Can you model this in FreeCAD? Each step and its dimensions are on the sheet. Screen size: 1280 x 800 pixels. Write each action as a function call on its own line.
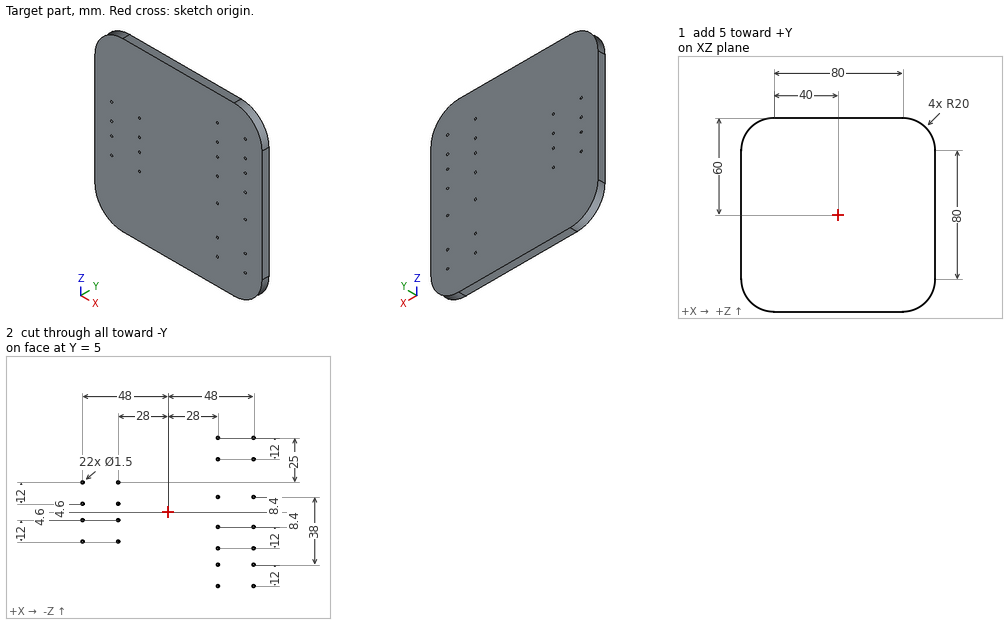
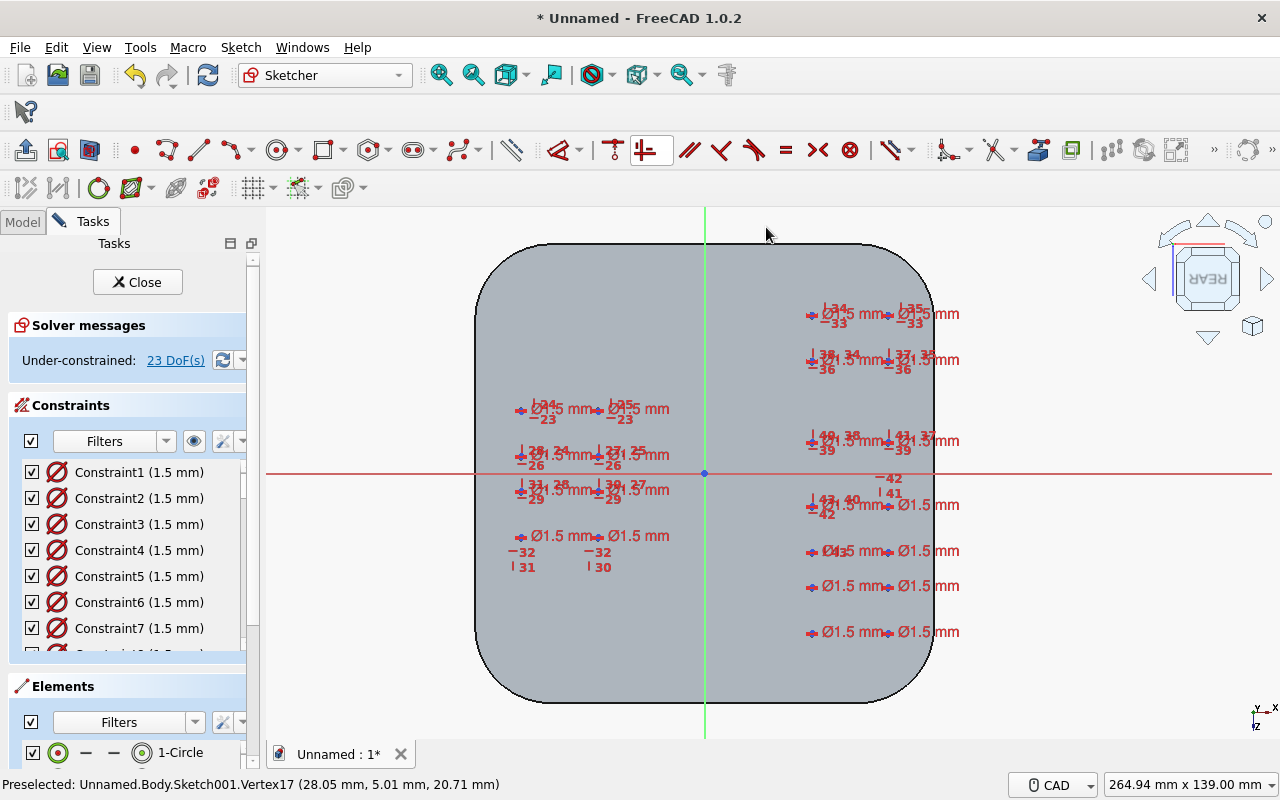
click(888, 507)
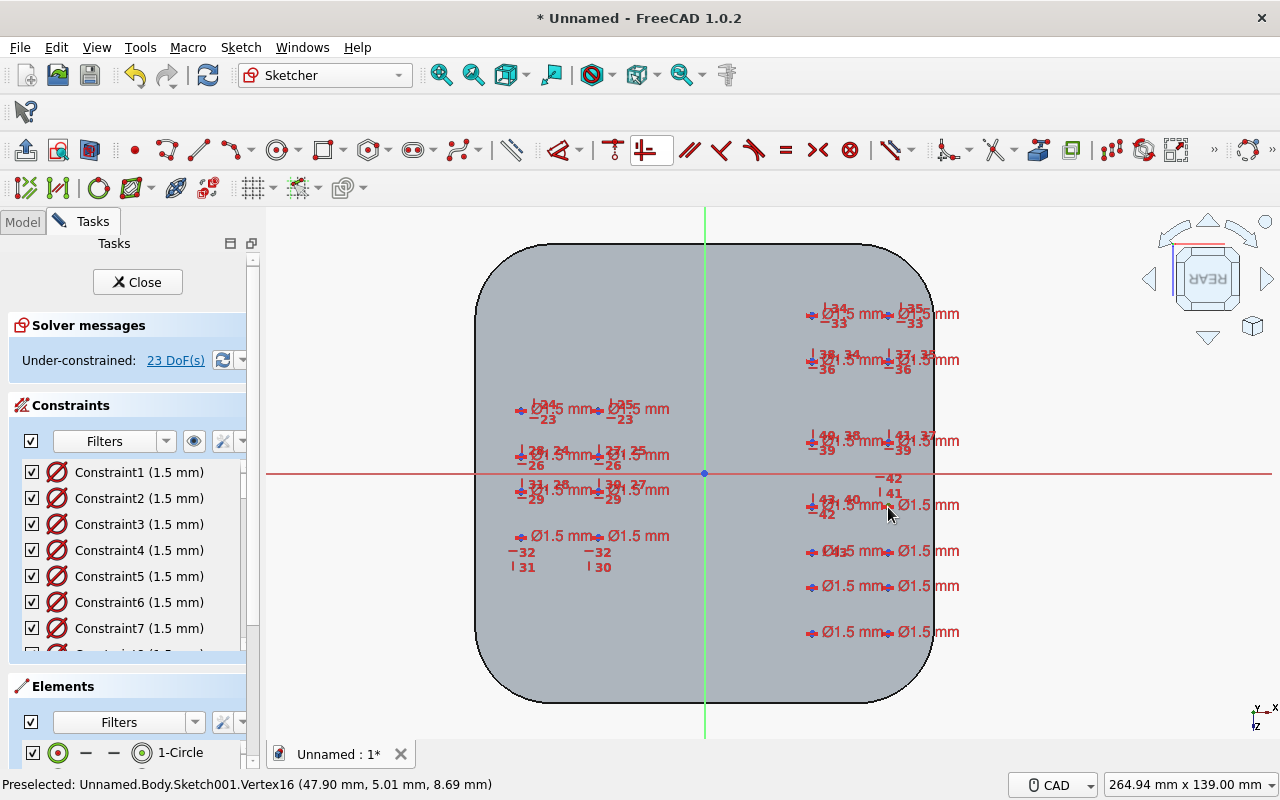
click(888, 553)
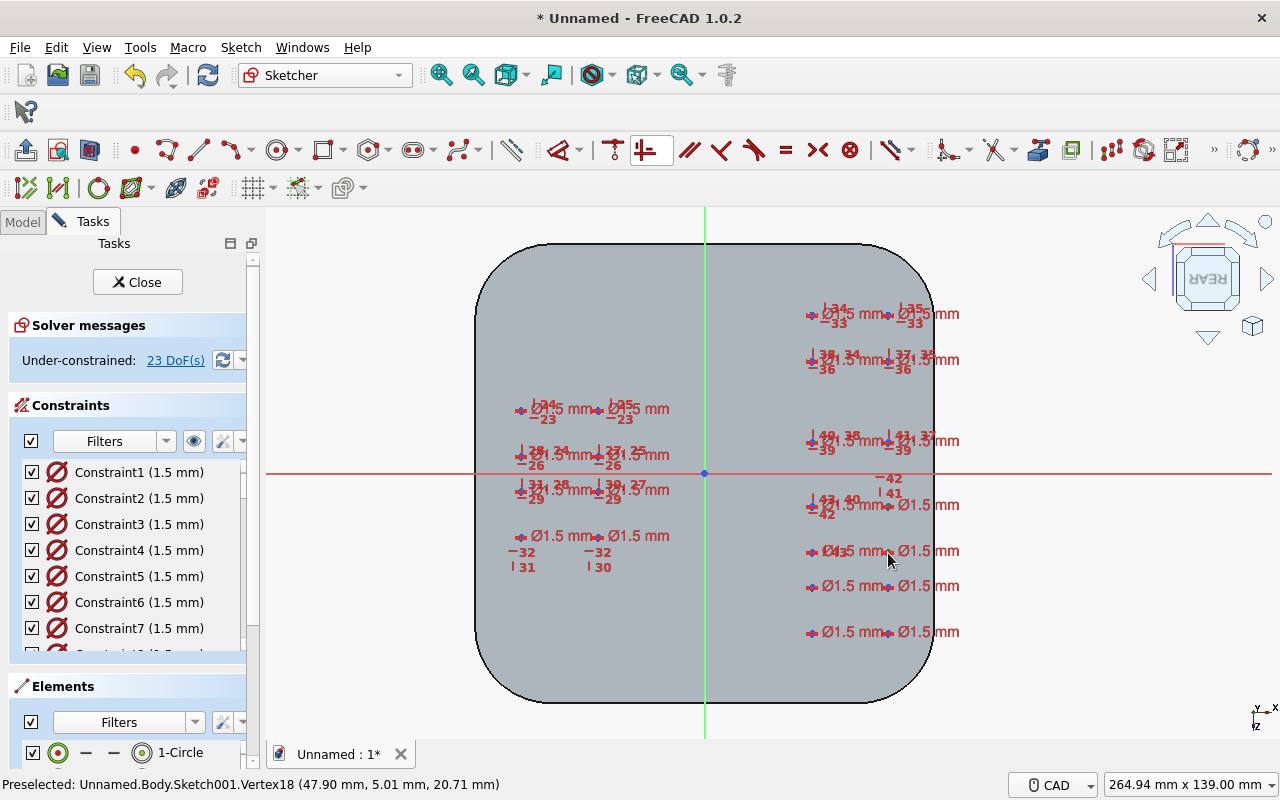
key(v)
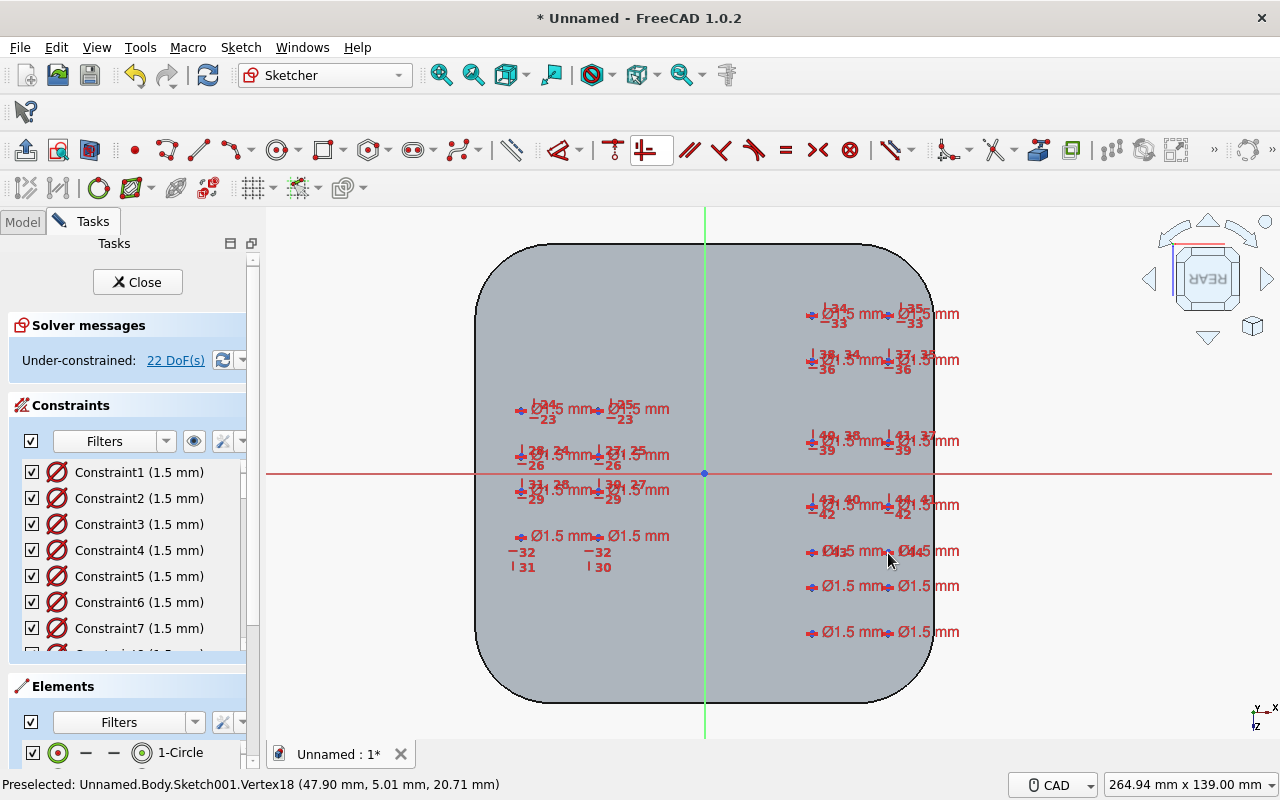
click(812, 553)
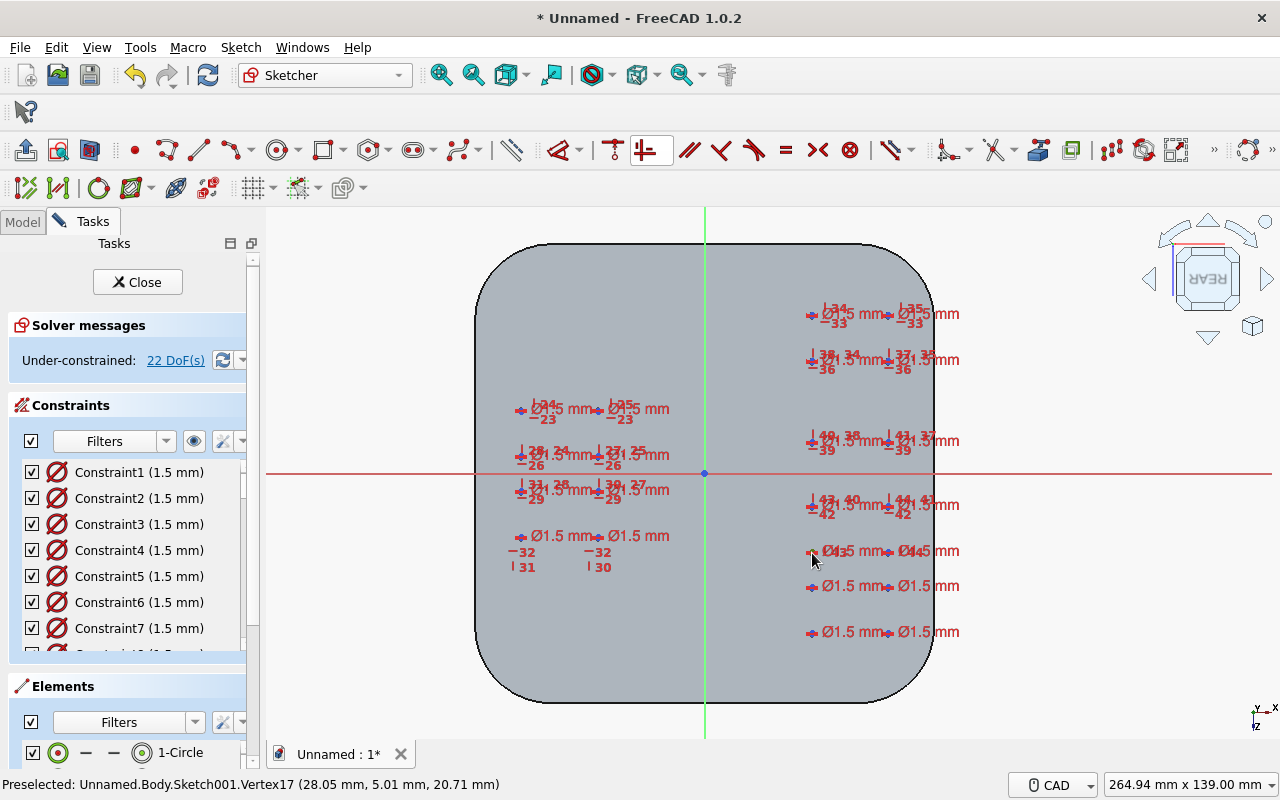
click(888, 553)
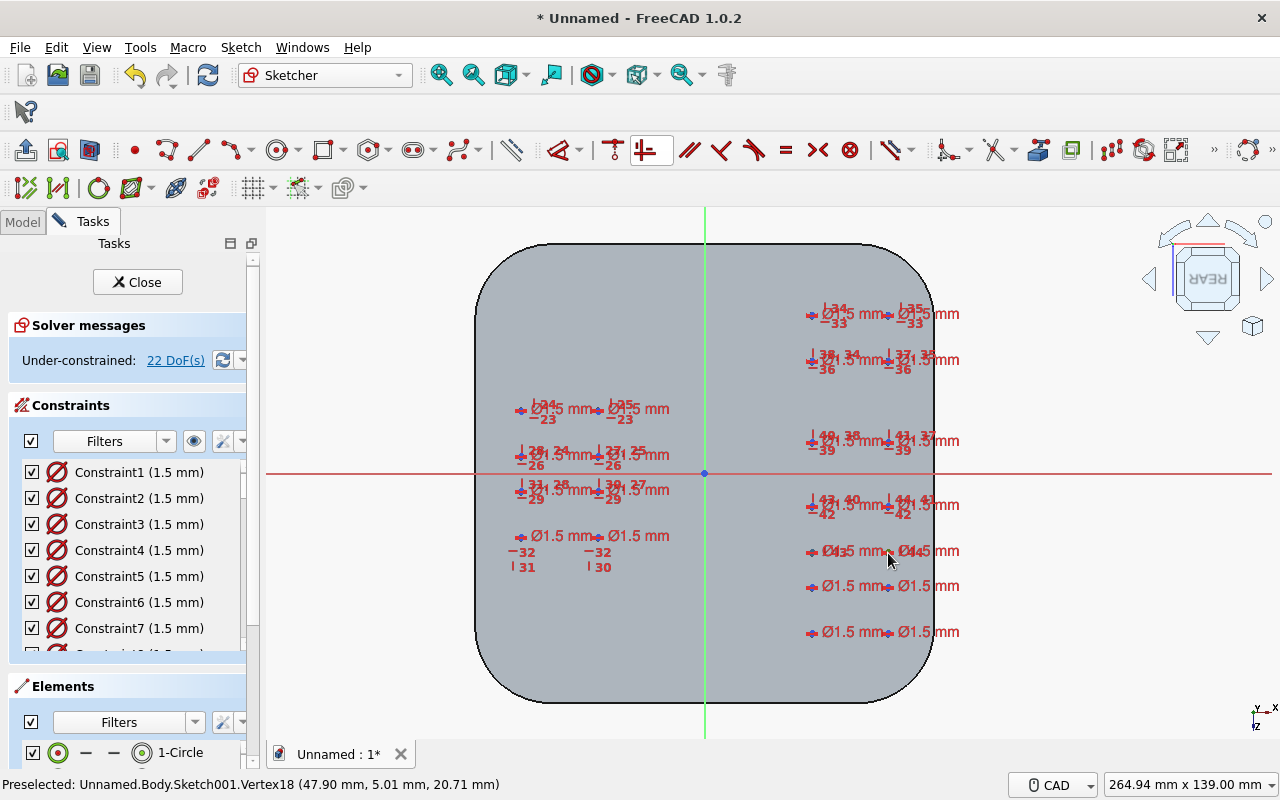
key(h)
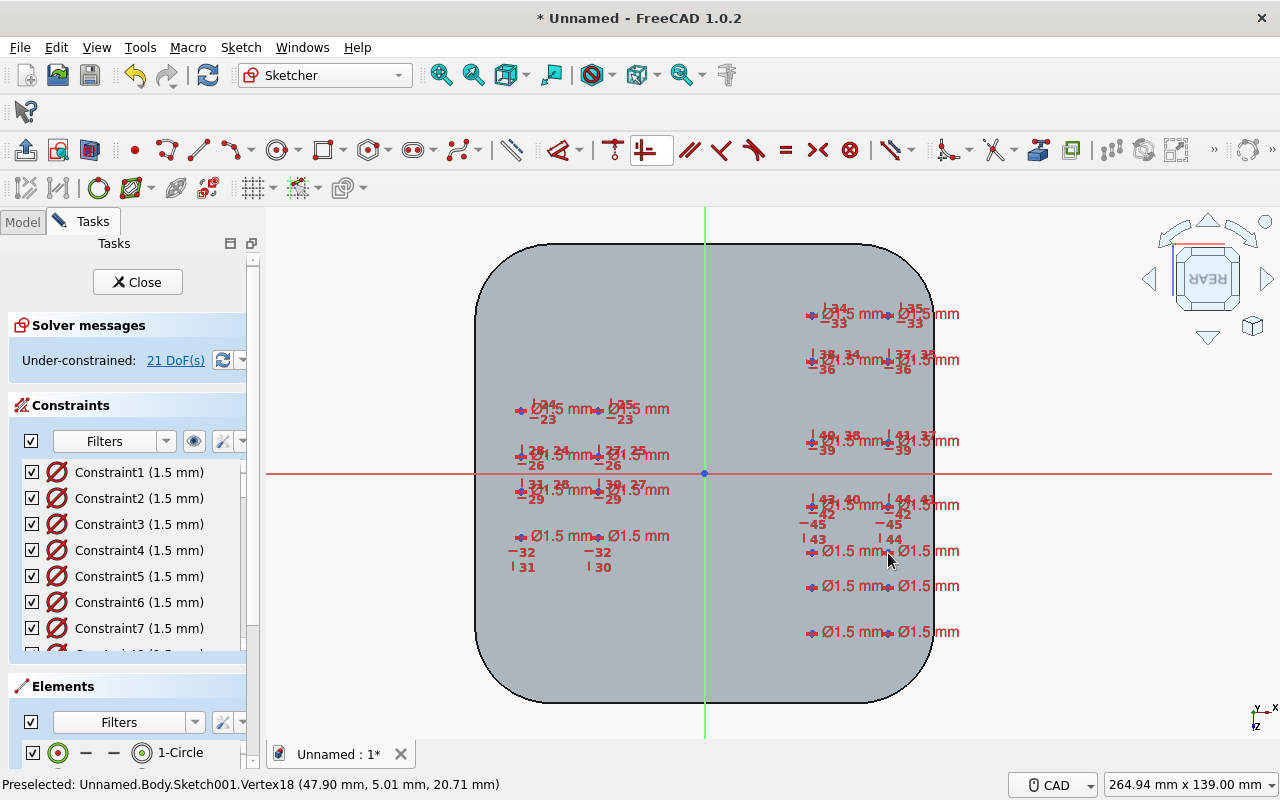
click(888, 553)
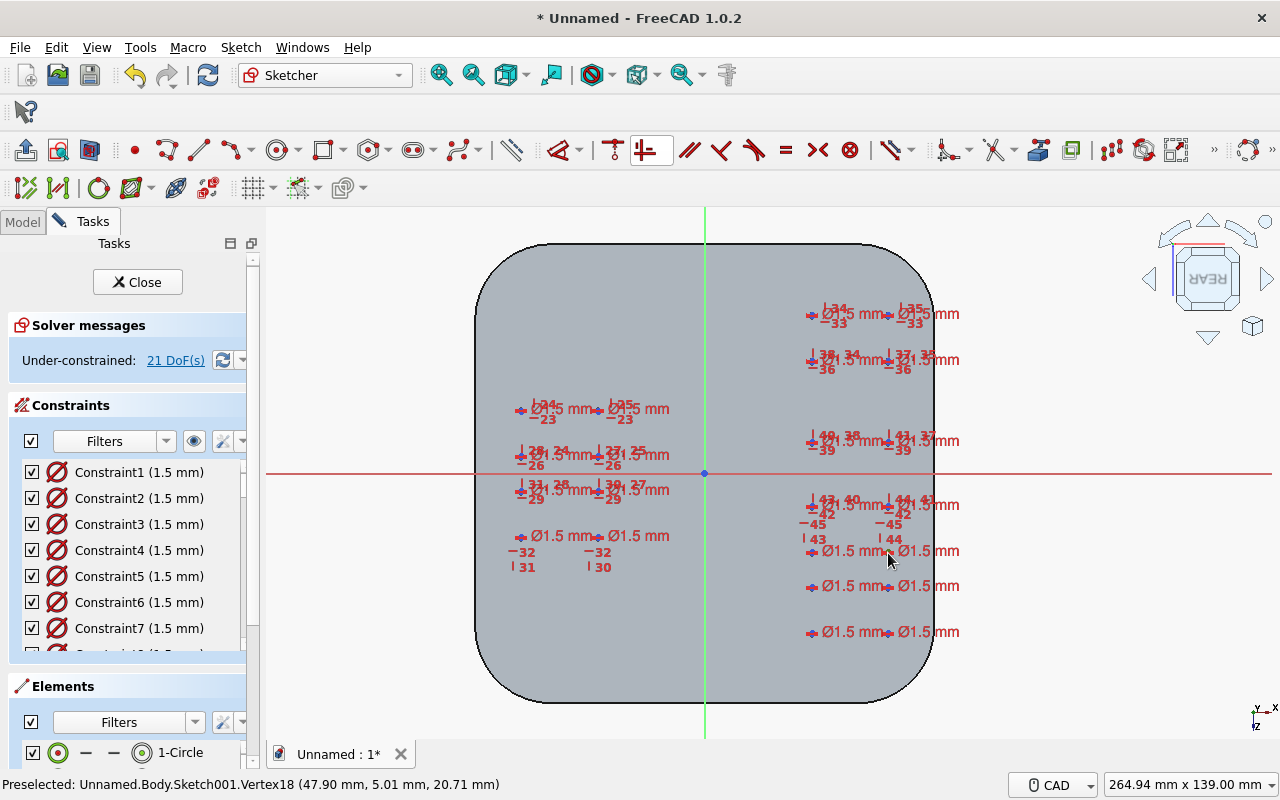
click(888, 588)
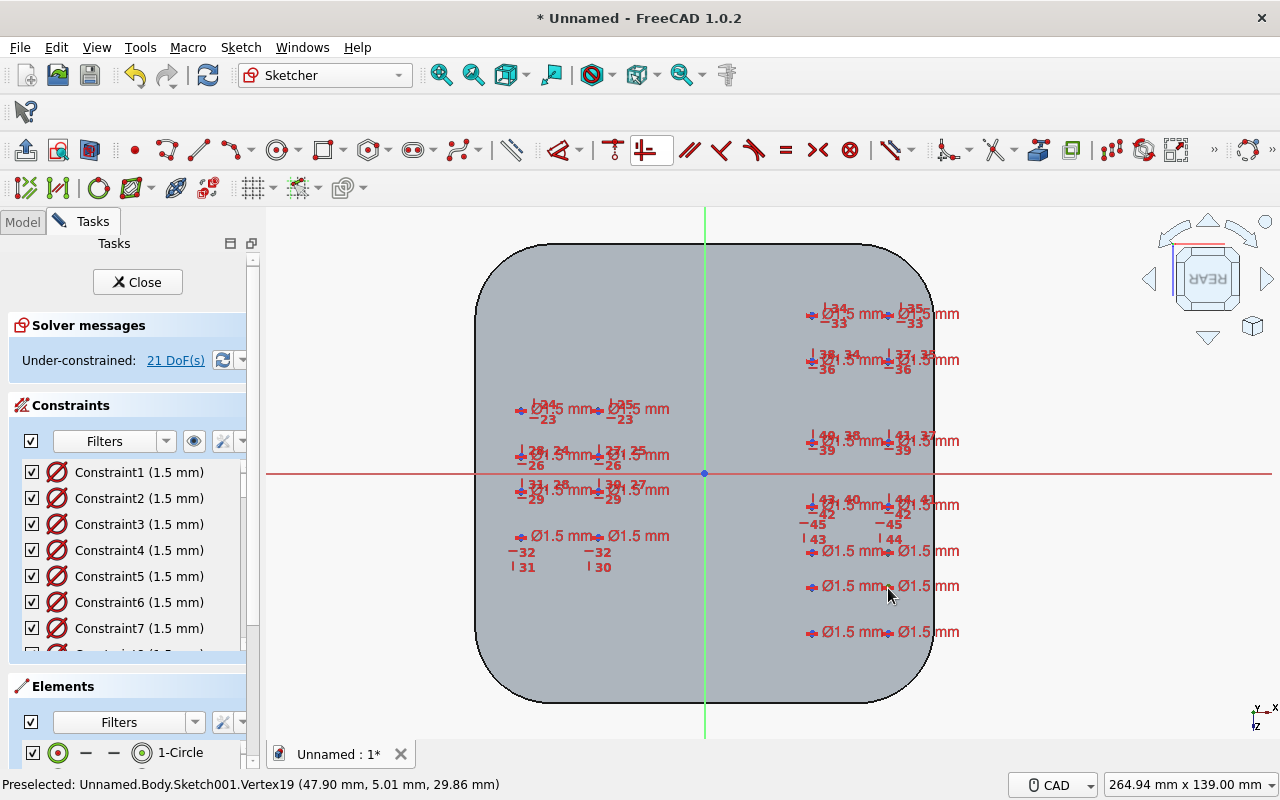
click(668, 150)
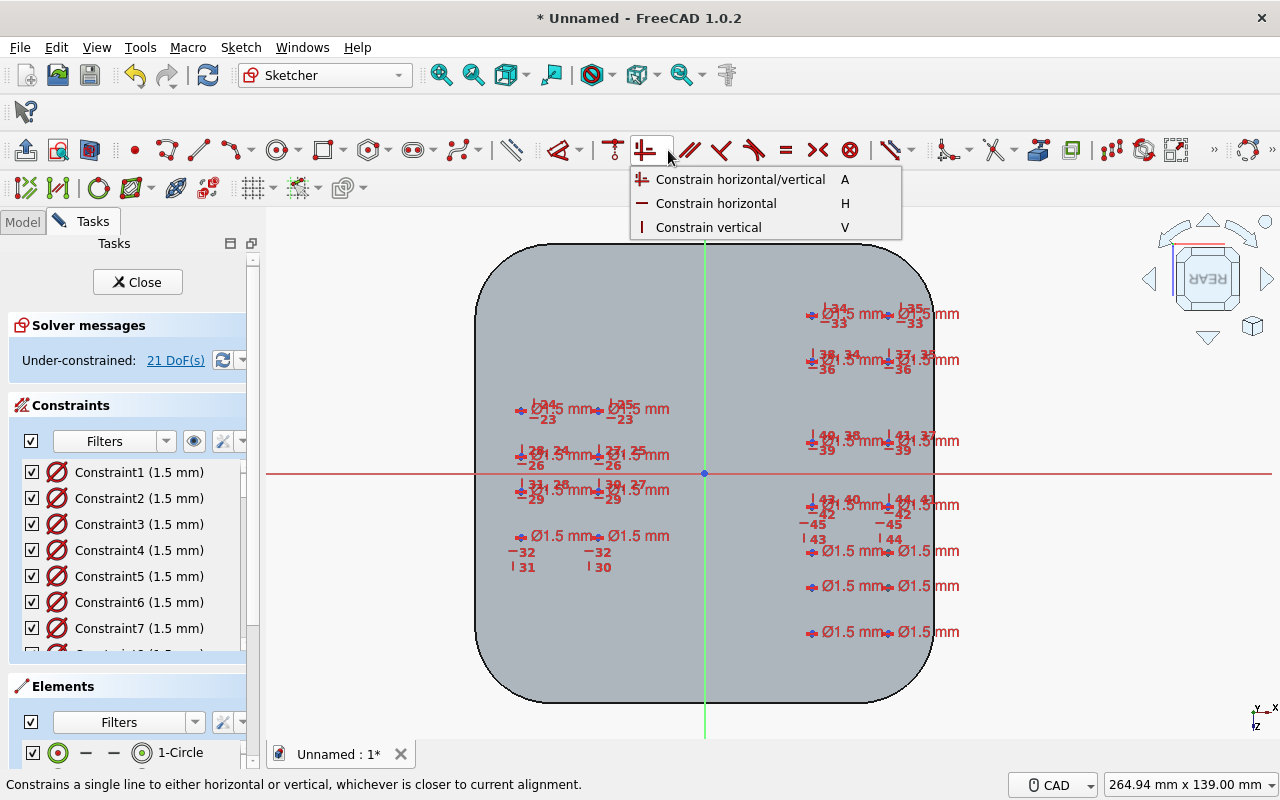
click(766, 227)